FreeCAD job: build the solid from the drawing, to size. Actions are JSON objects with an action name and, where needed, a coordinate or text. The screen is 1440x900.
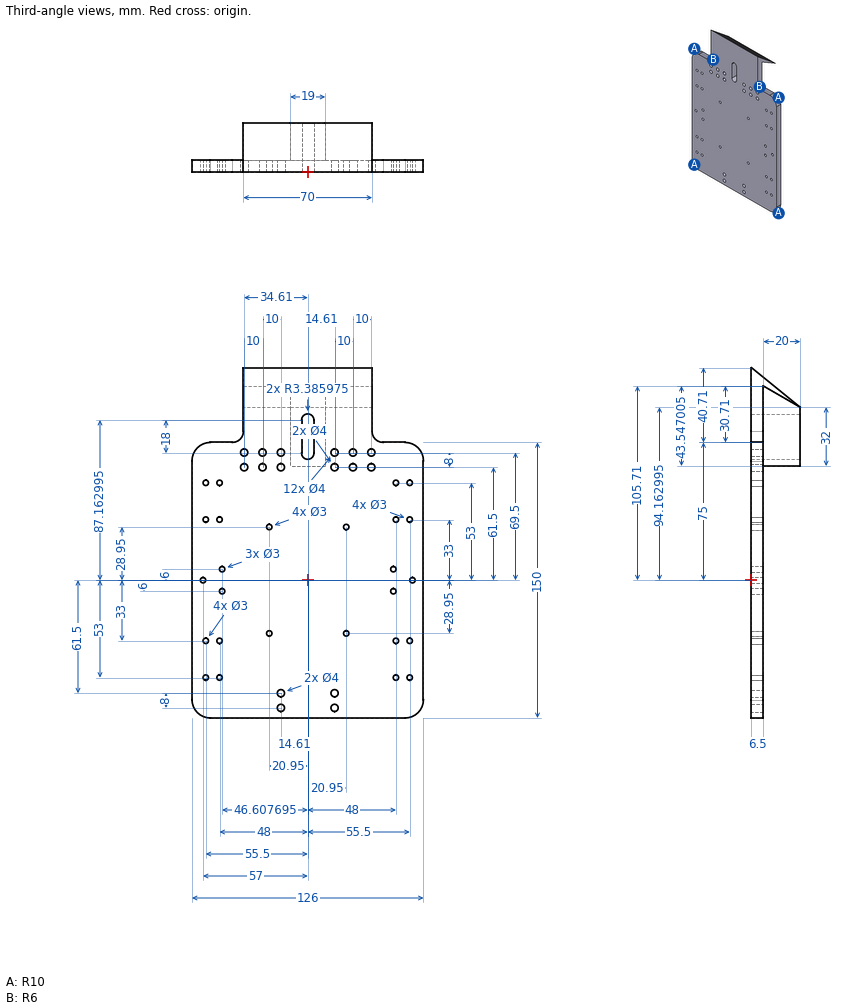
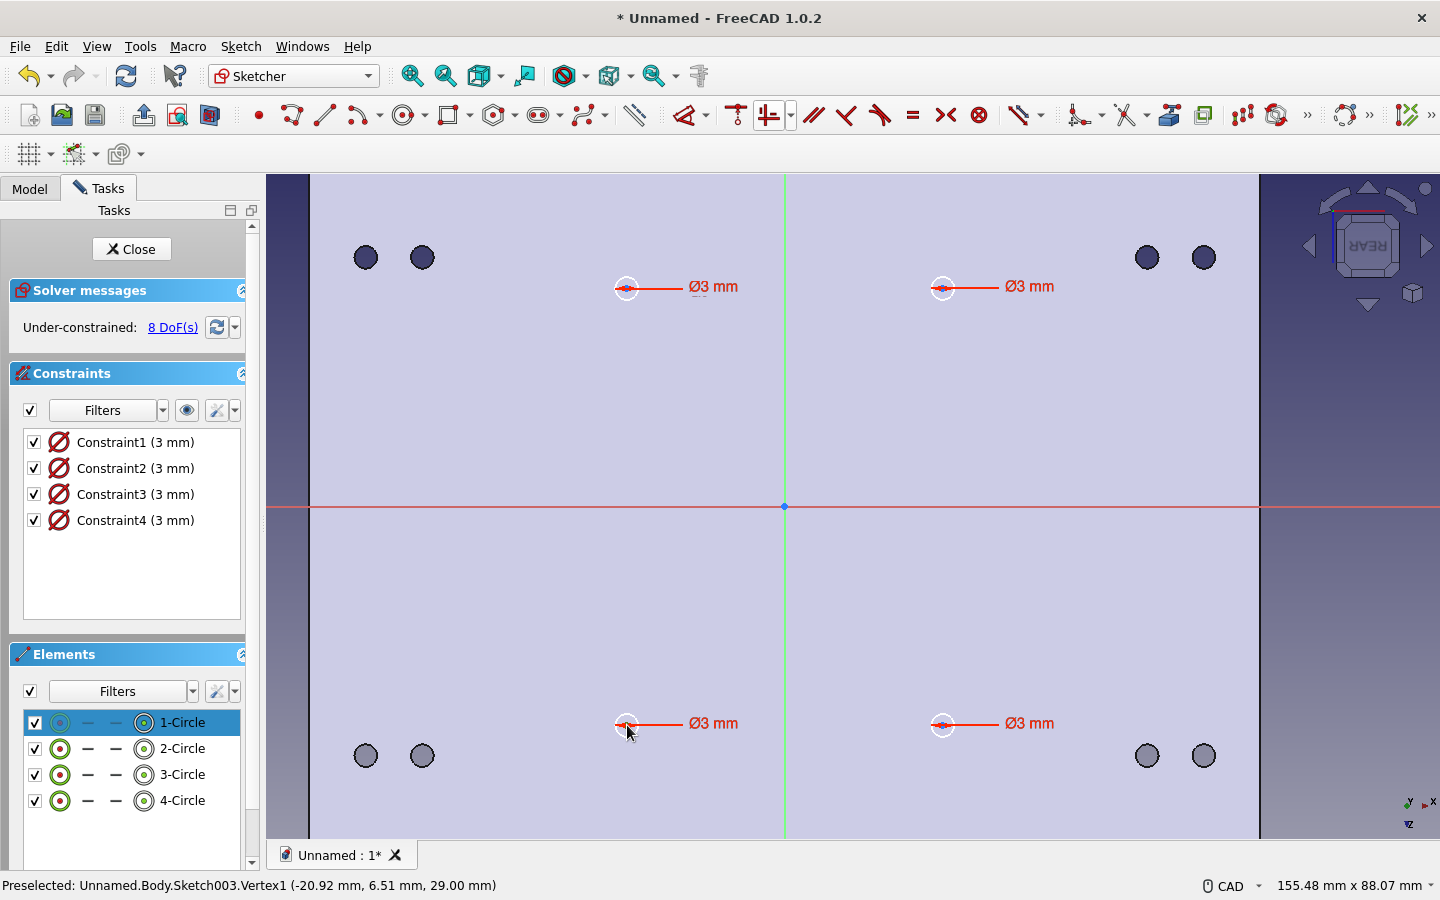
{"action": "left_click", "coordinate": [943, 725]}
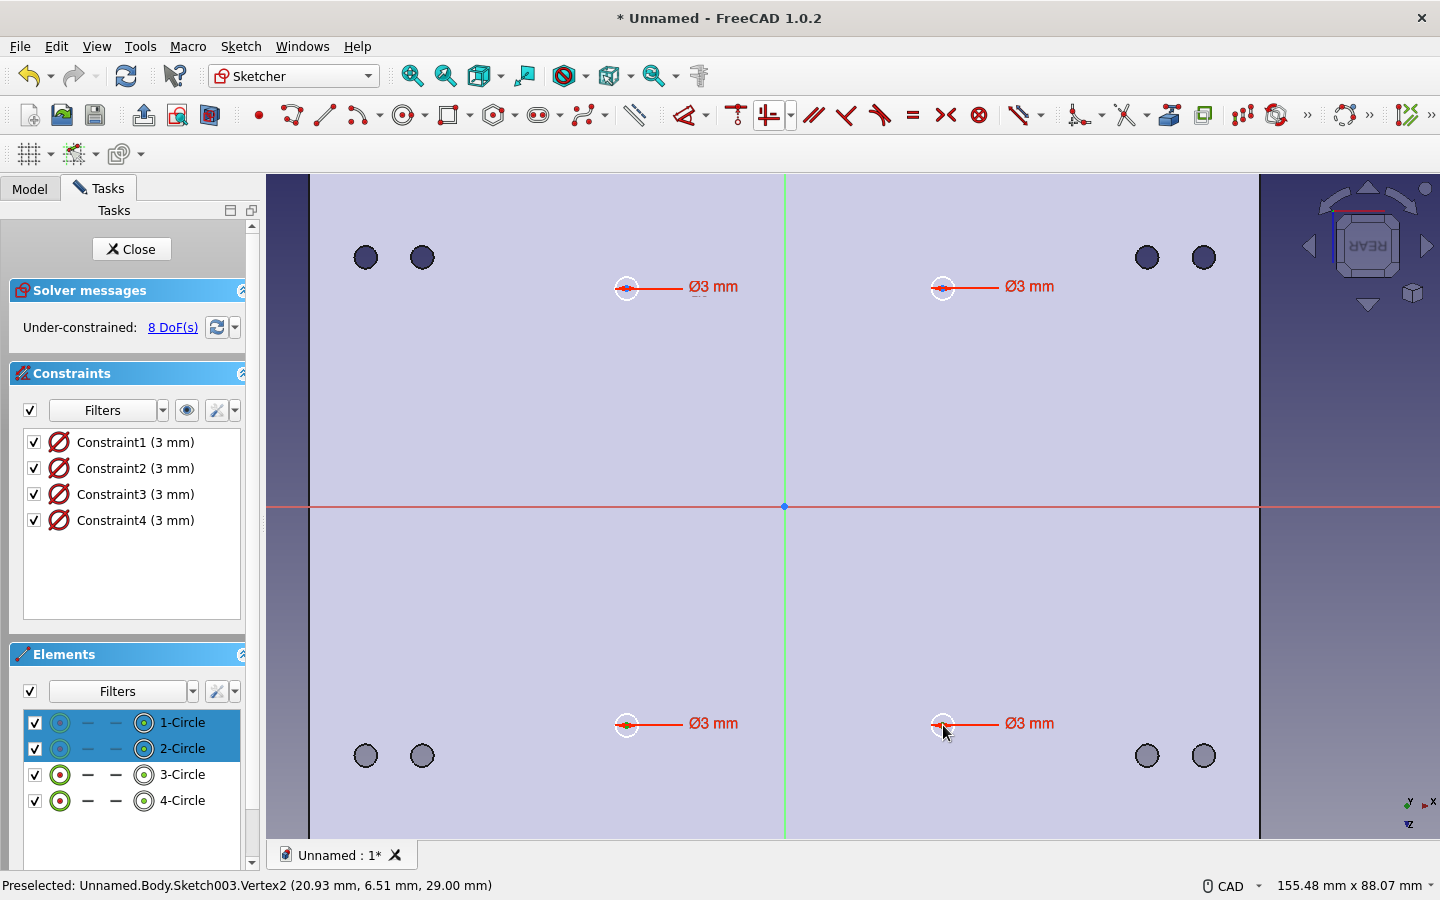
{"action": "left_click", "coordinate": [790, 116]}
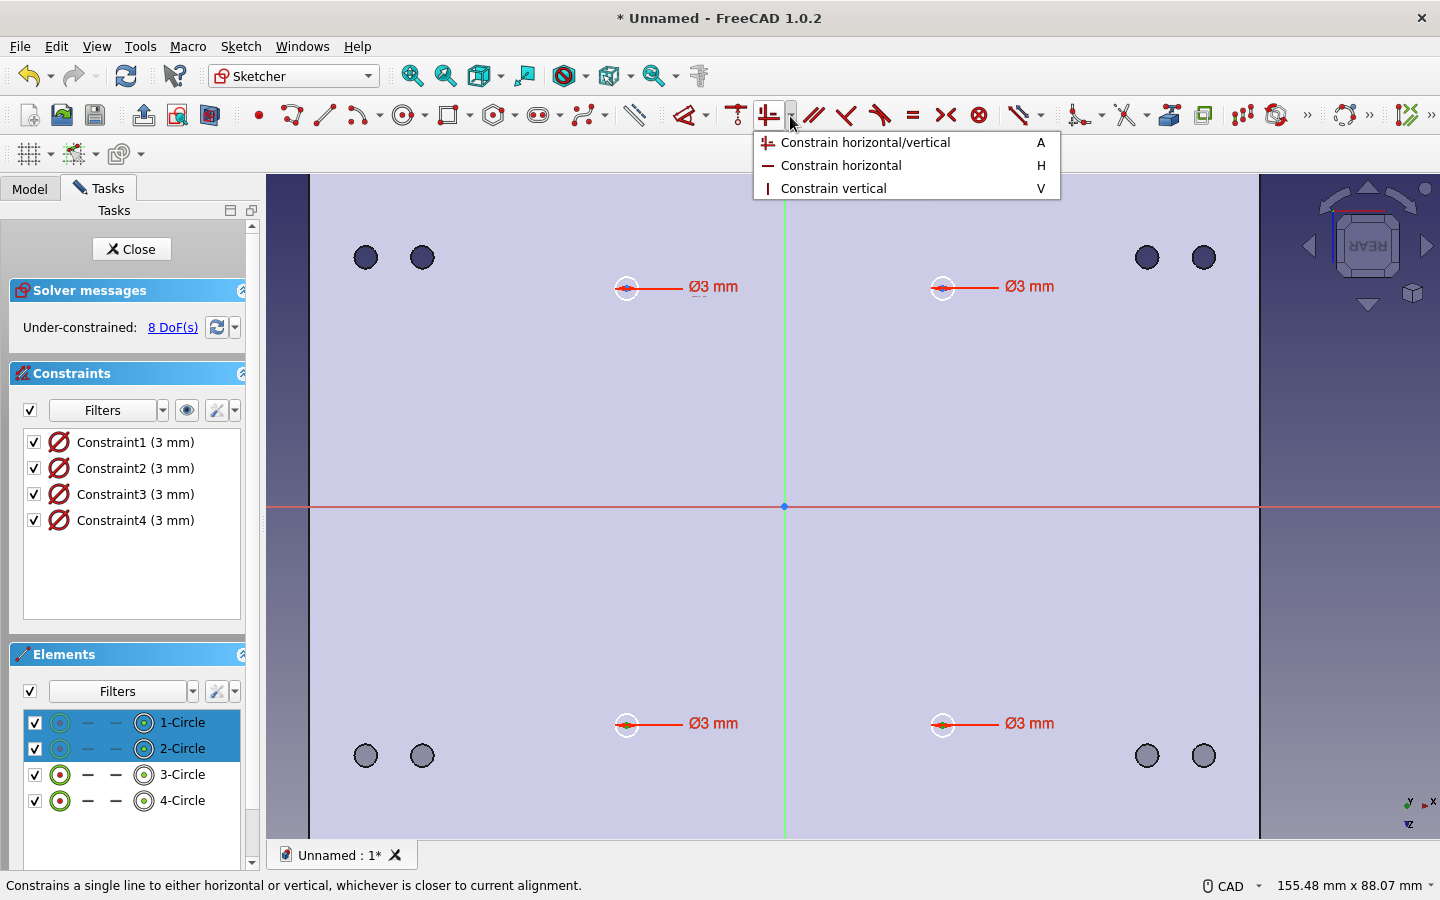
{"action": "left_click", "coordinate": [907, 166]}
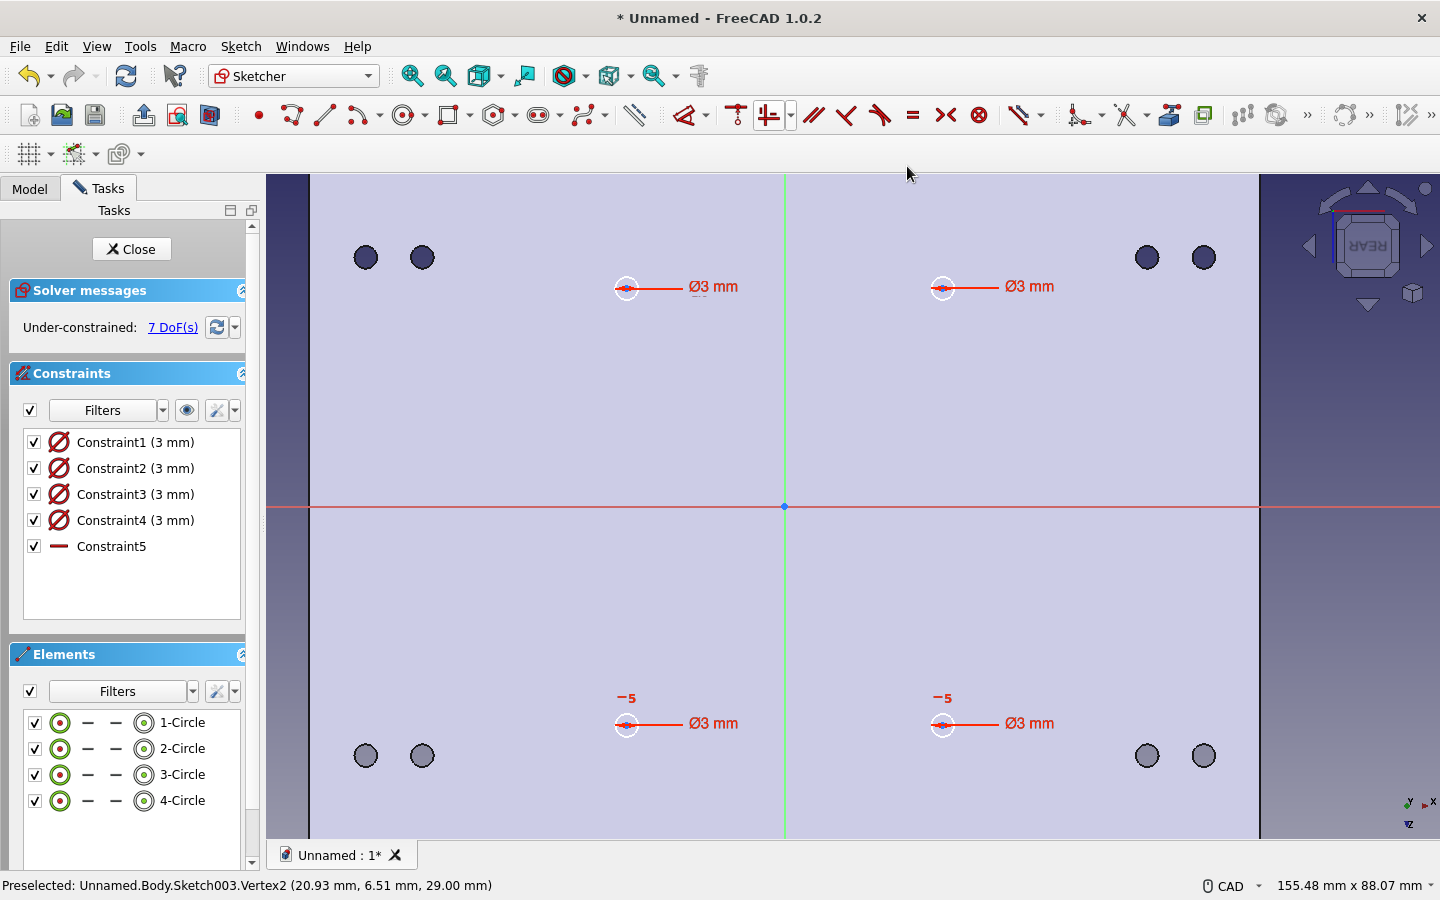
{"action": "left_click", "coordinate": [943, 725]}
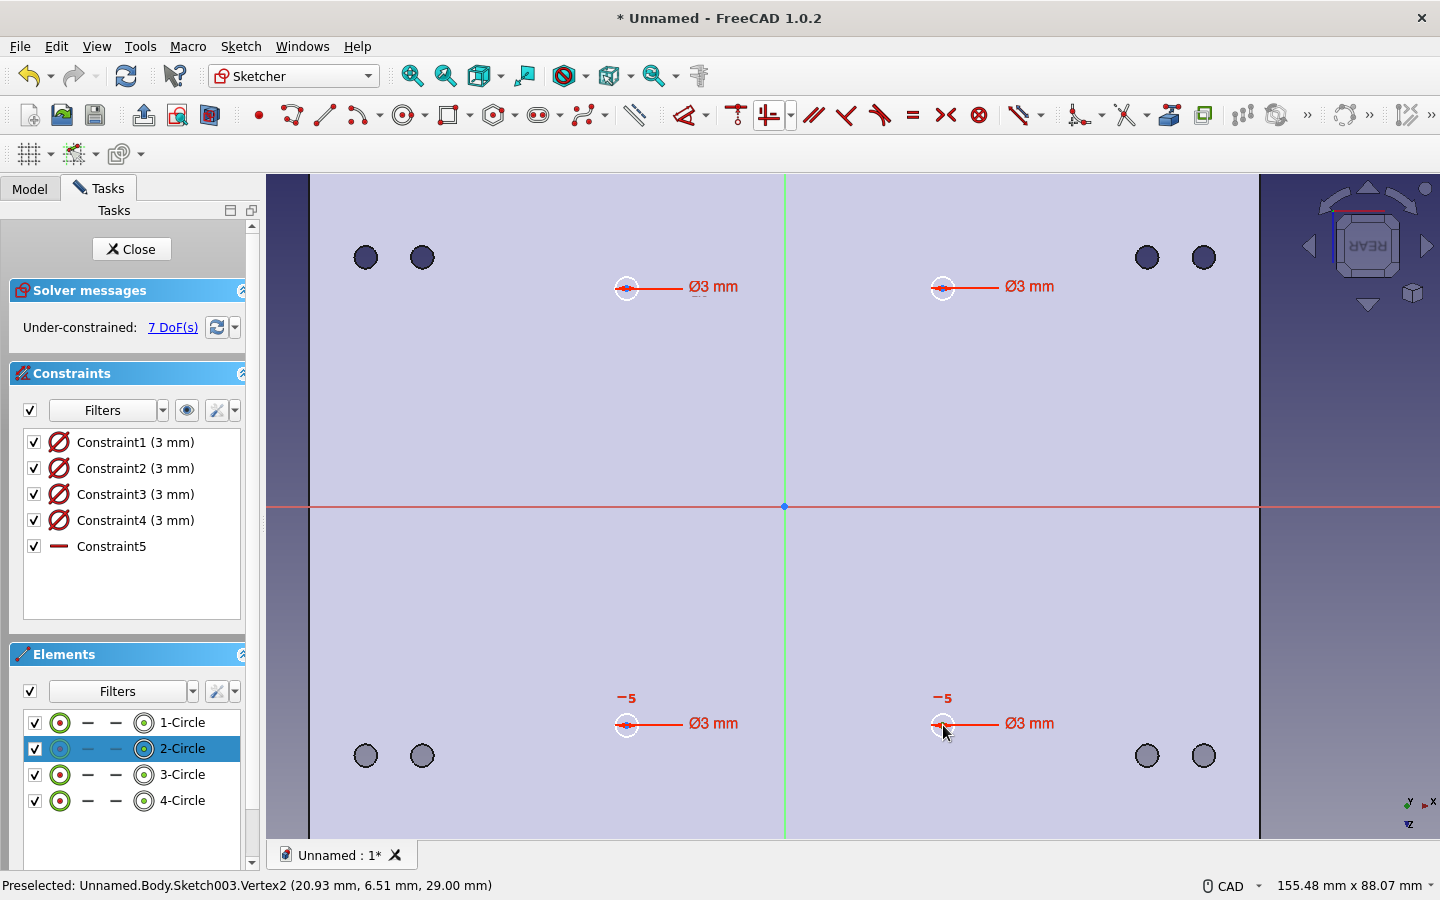
{"action": "left_click", "coordinate": [943, 288]}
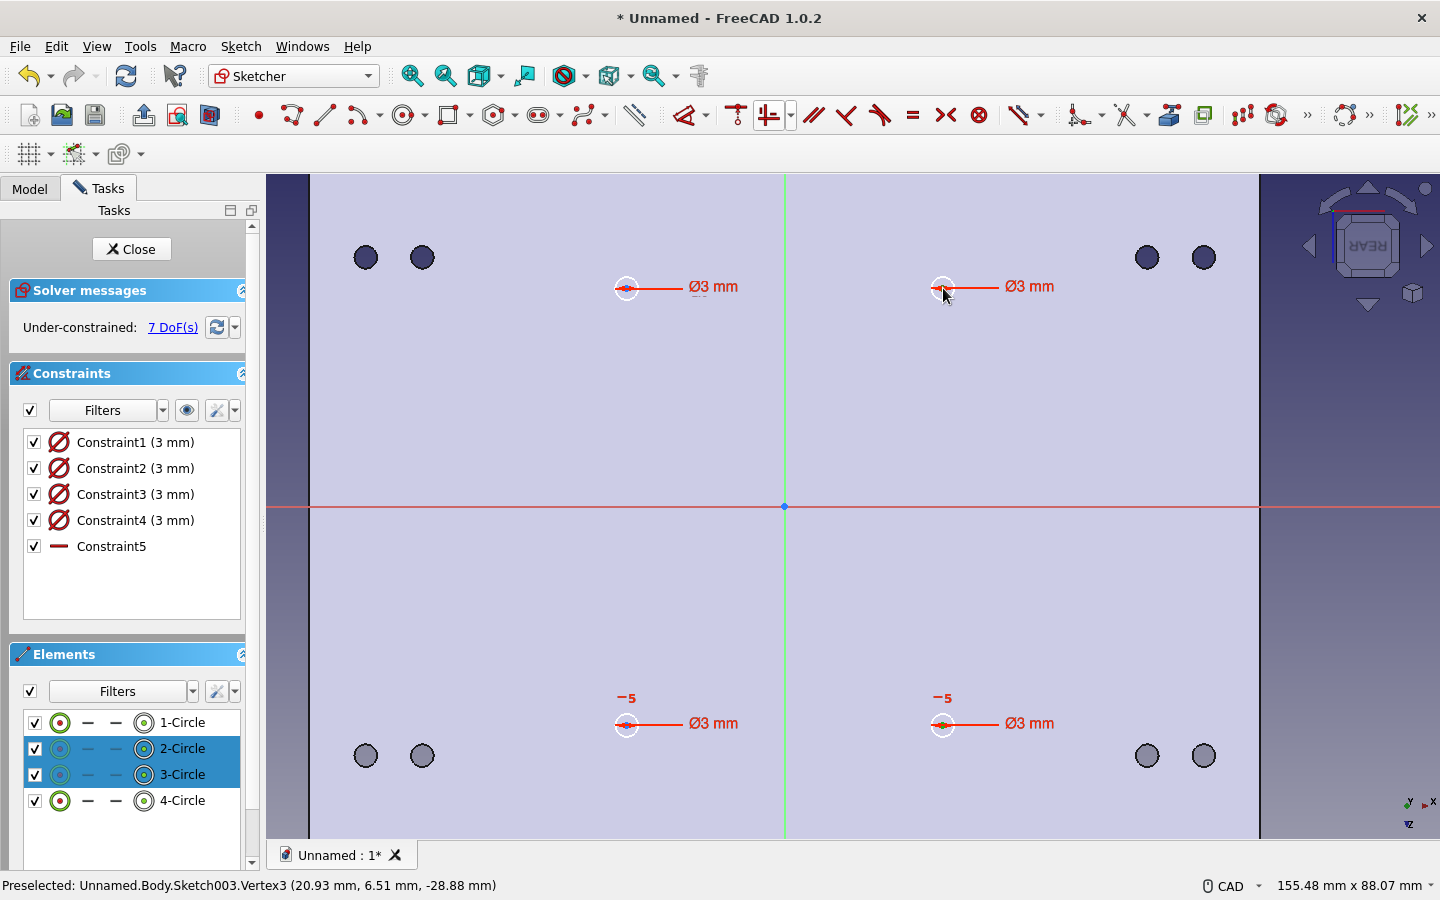
{"action": "key", "text": "v"}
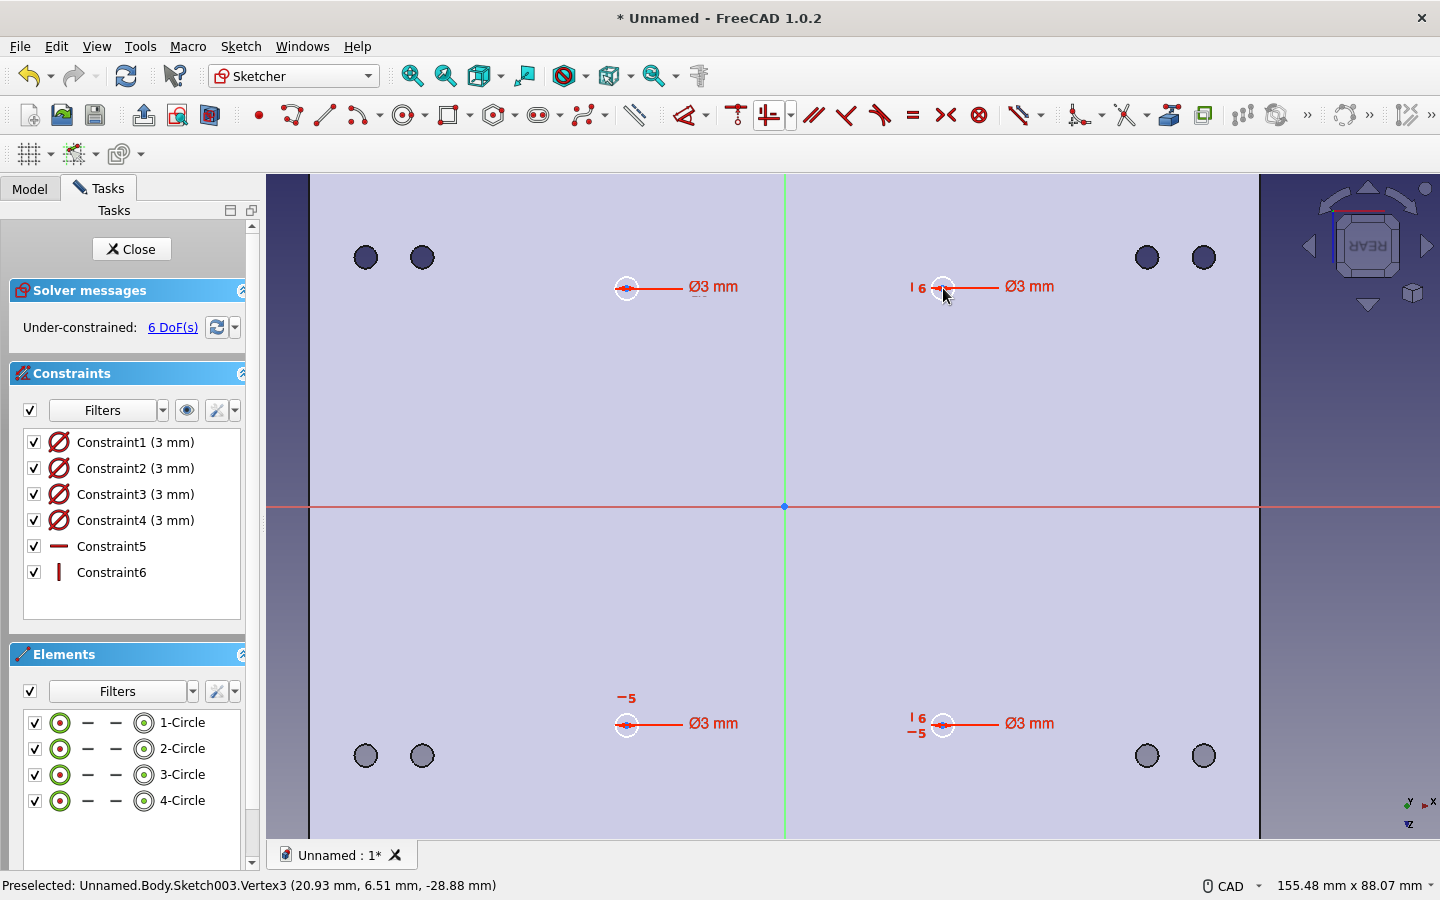
{"action": "left_click", "coordinate": [627, 725]}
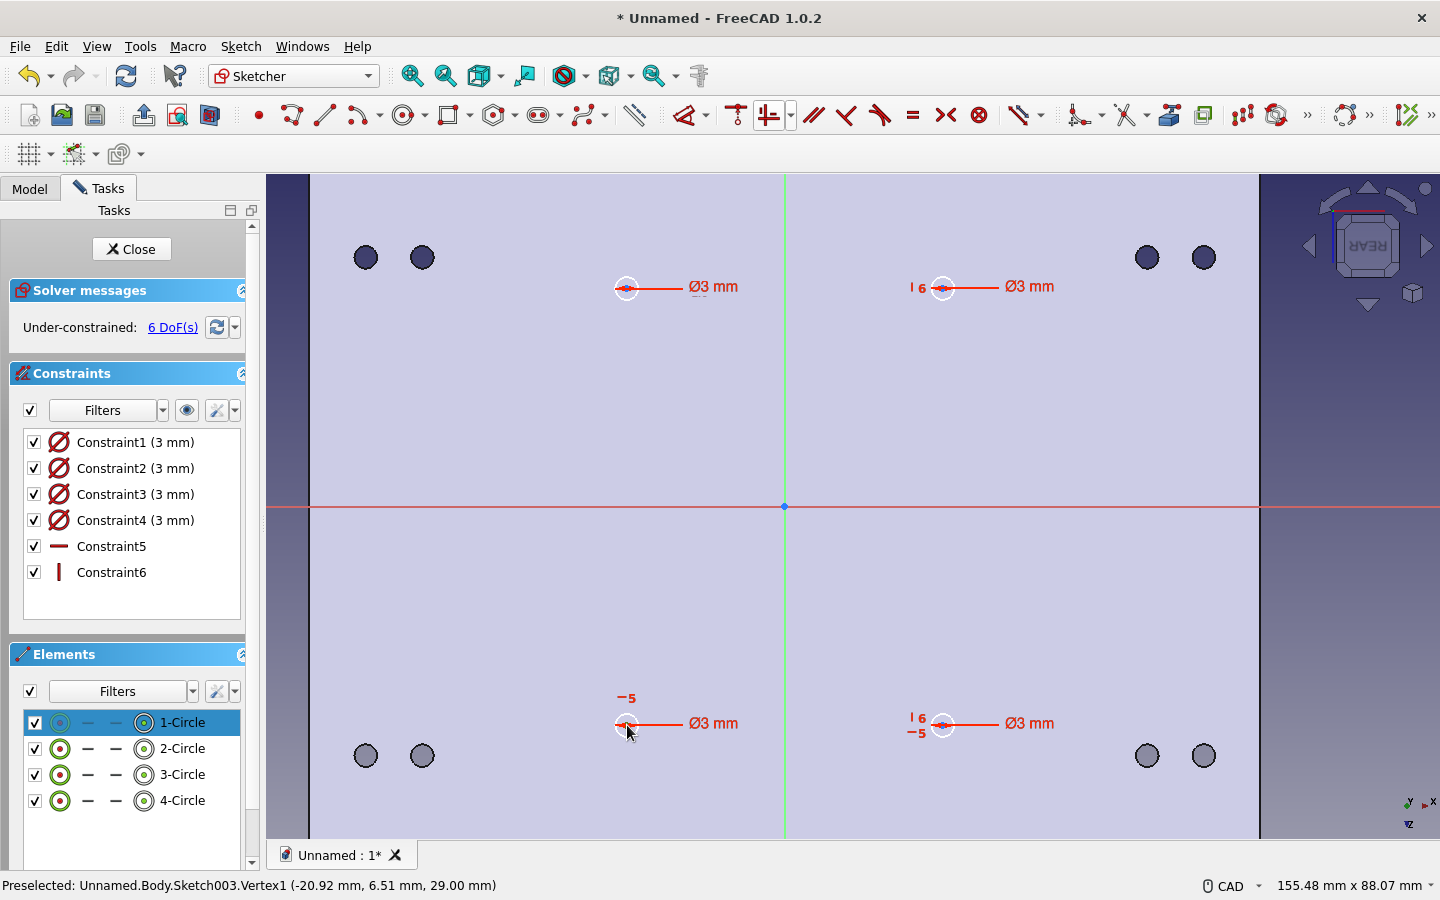
{"action": "left_click", "coordinate": [627, 289]}